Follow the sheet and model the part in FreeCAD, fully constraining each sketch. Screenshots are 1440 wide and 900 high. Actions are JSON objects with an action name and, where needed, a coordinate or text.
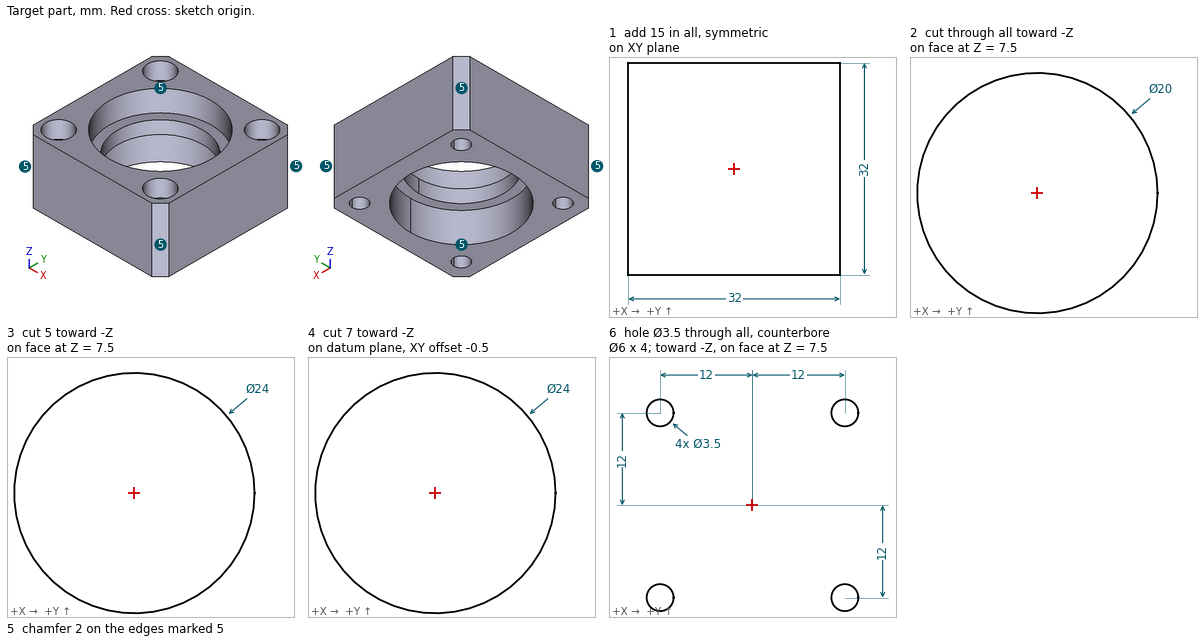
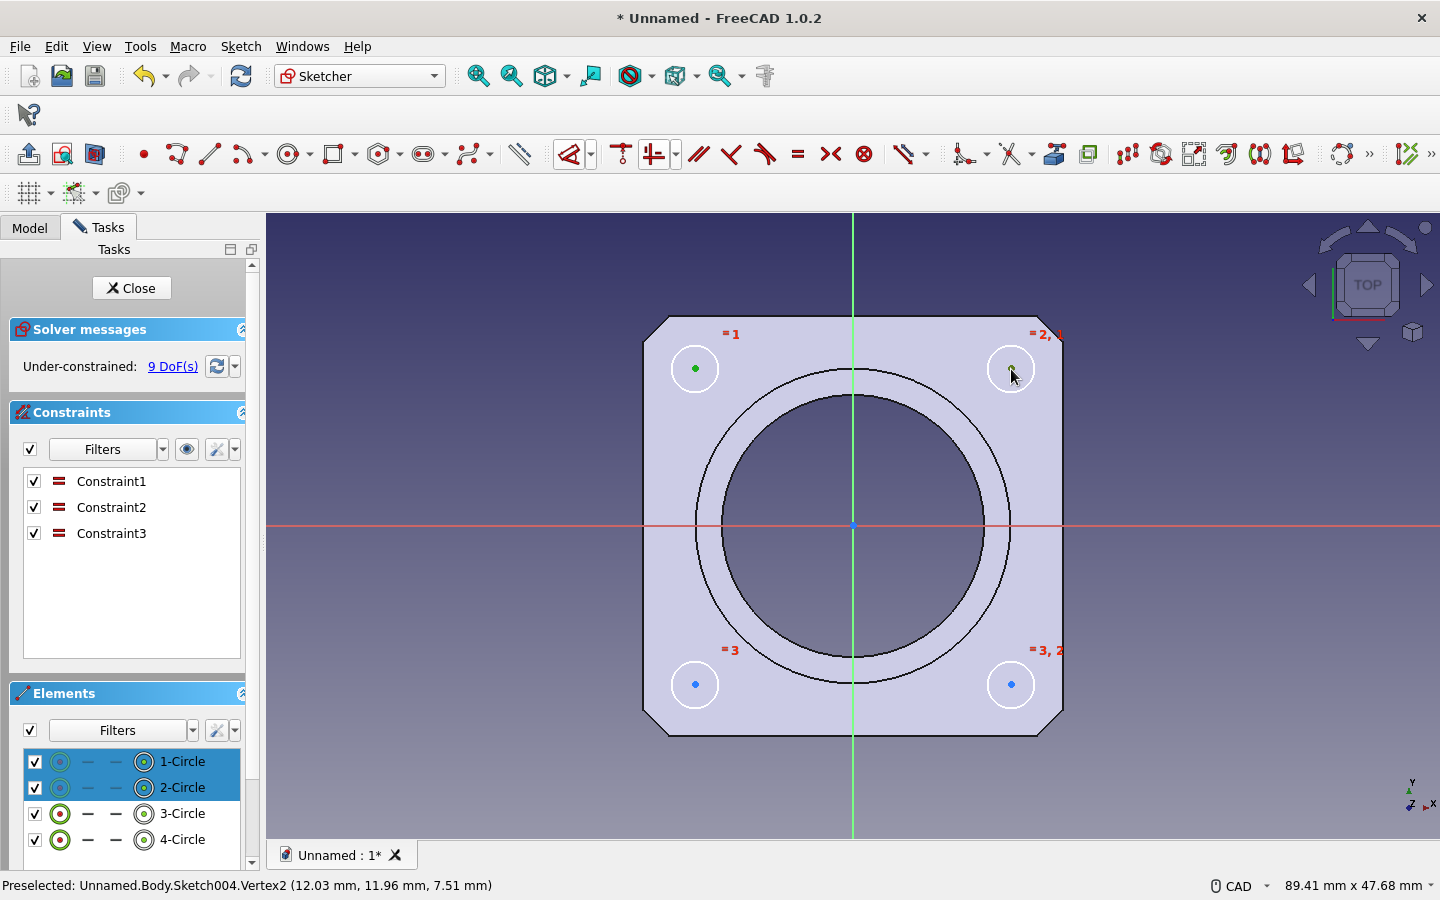
{"action": "key", "text": "h"}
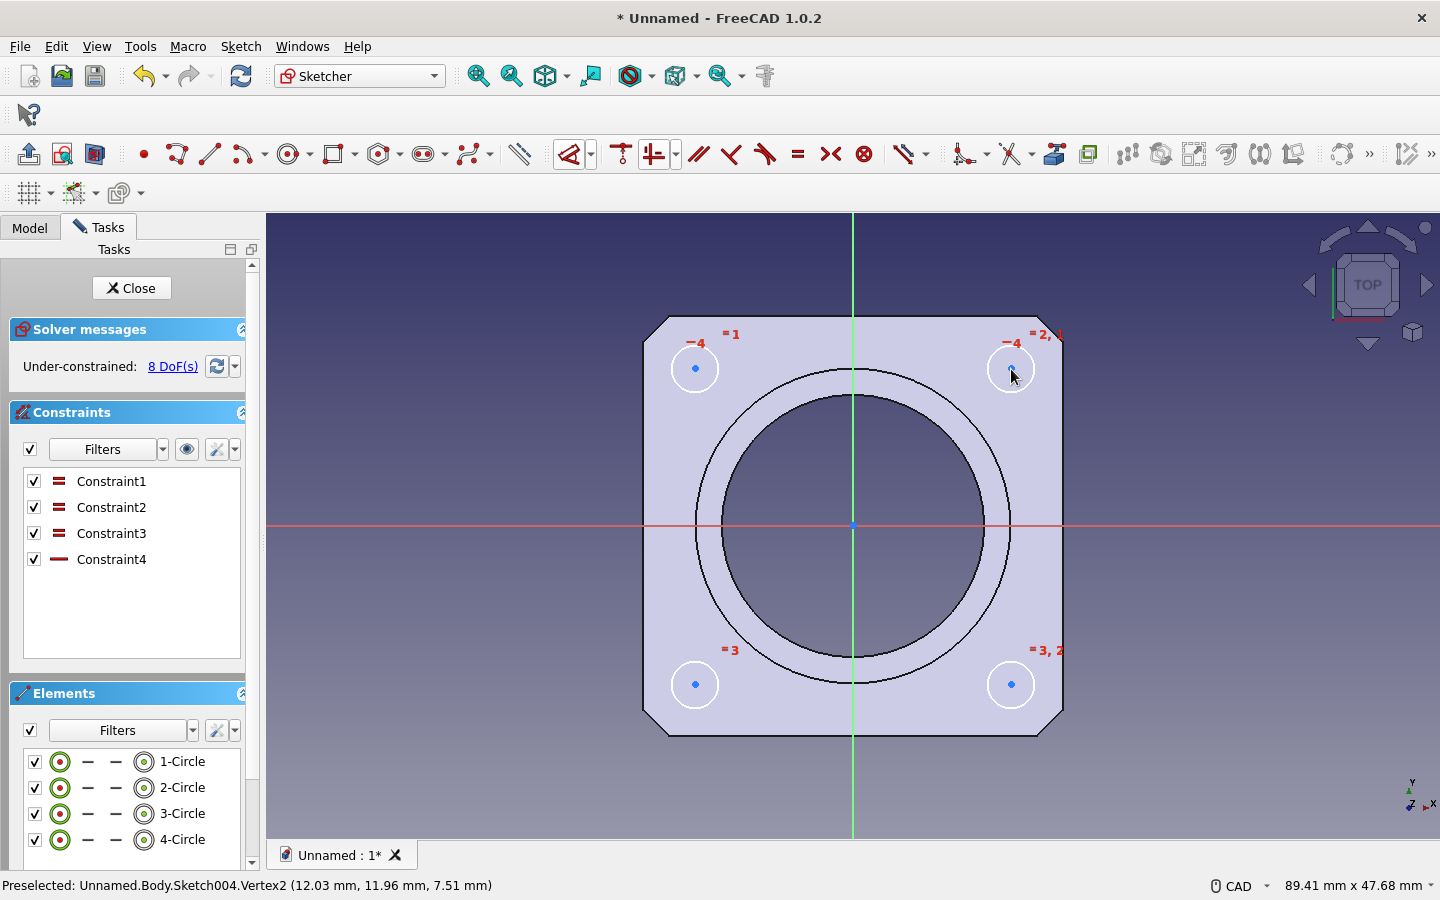
{"action": "left_click", "coordinate": [1011, 369]}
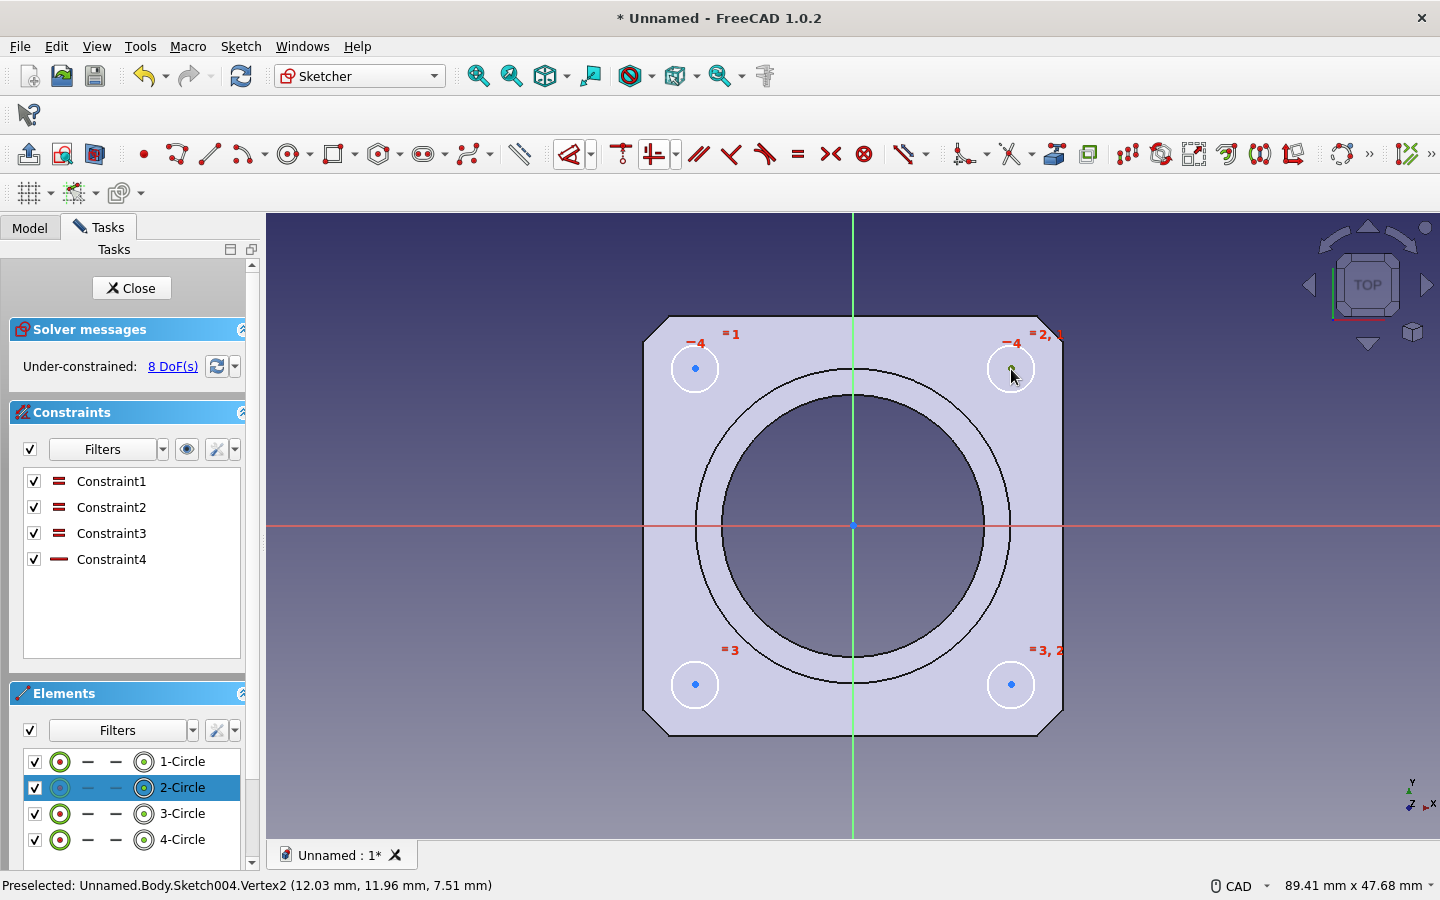
{"action": "left_click", "coordinate": [1011, 685]}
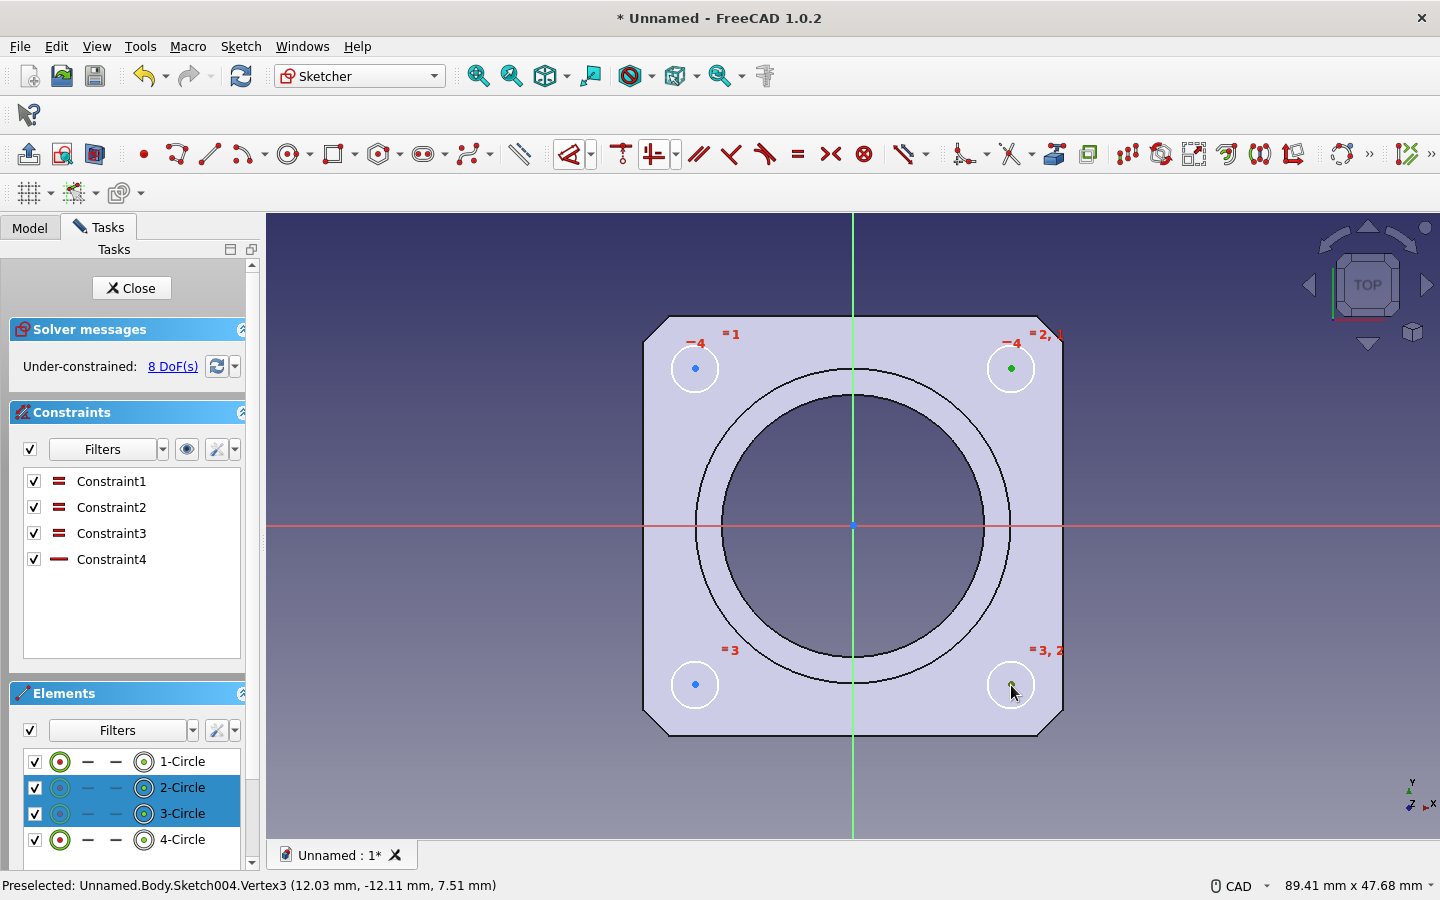
{"action": "key", "text": "v"}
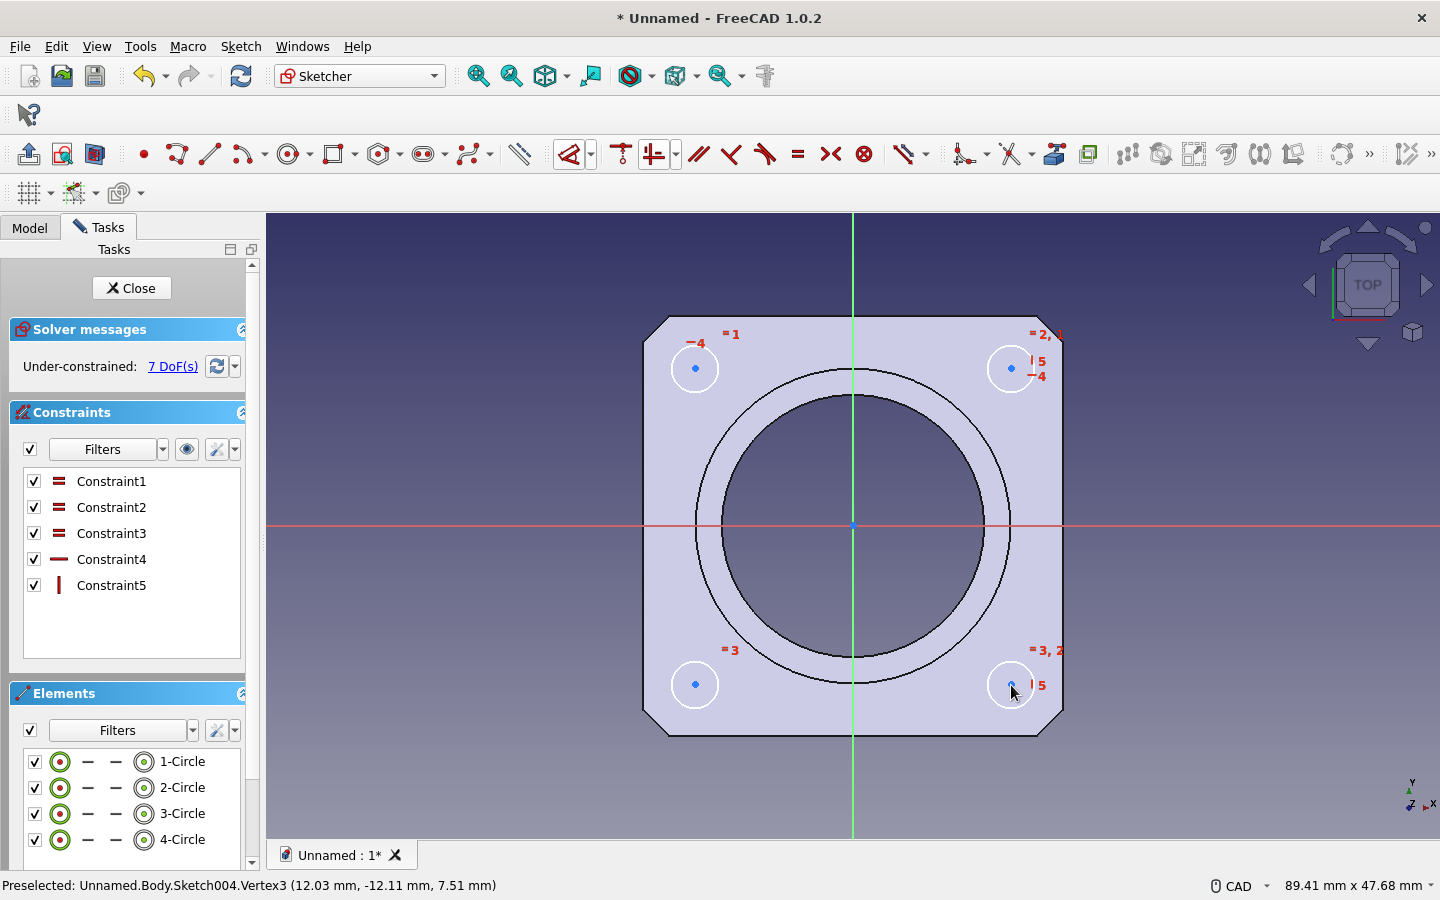
{"action": "left_click", "coordinate": [695, 369]}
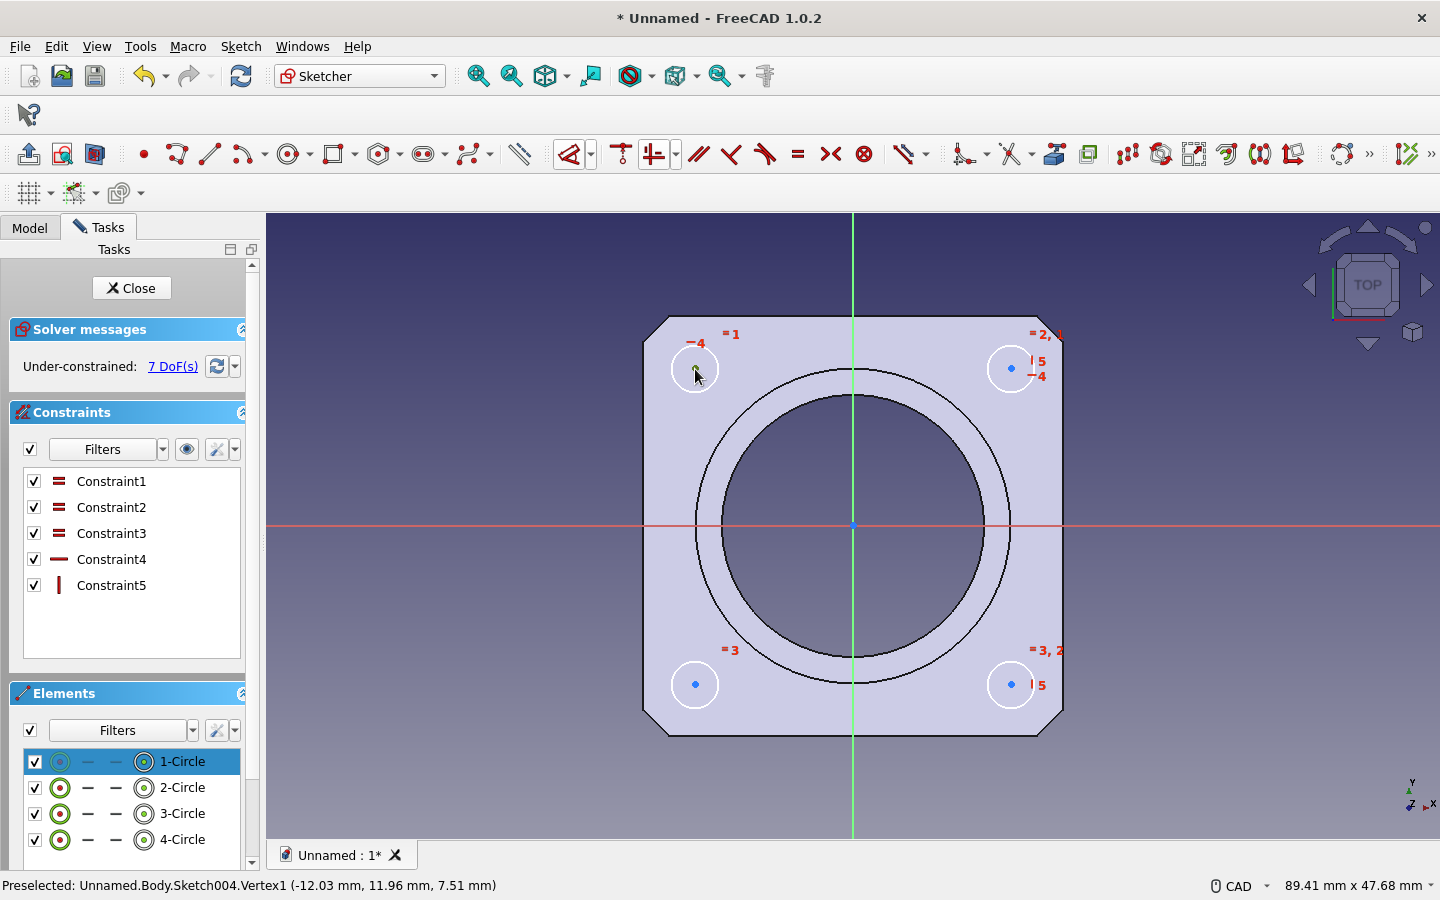
{"action": "left_click", "coordinate": [695, 685]}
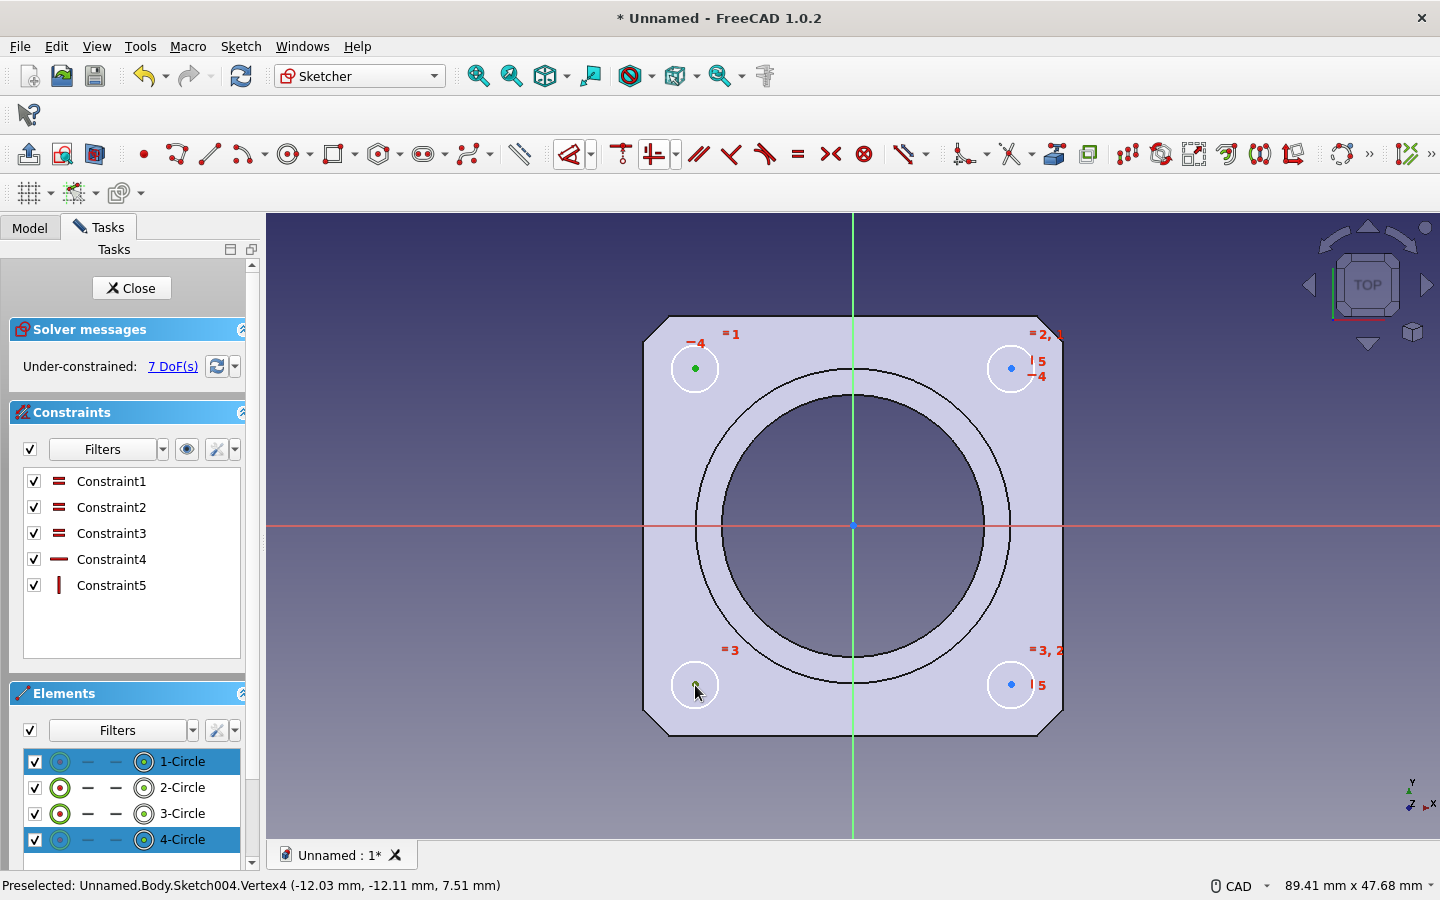
{"action": "left_click", "coordinate": [676, 154]}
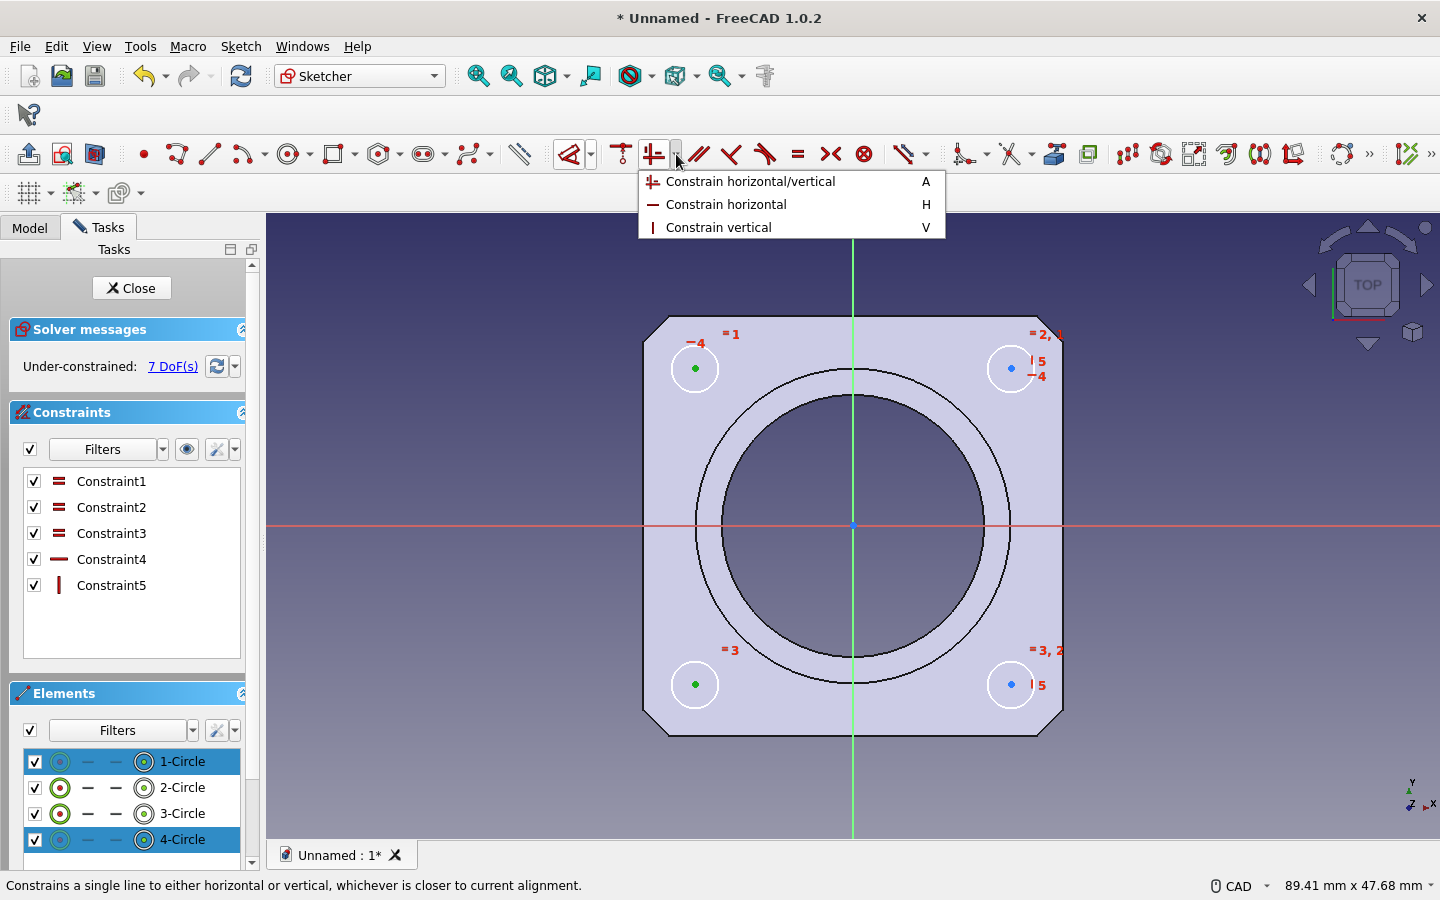
{"action": "left_click", "coordinate": [792, 228]}